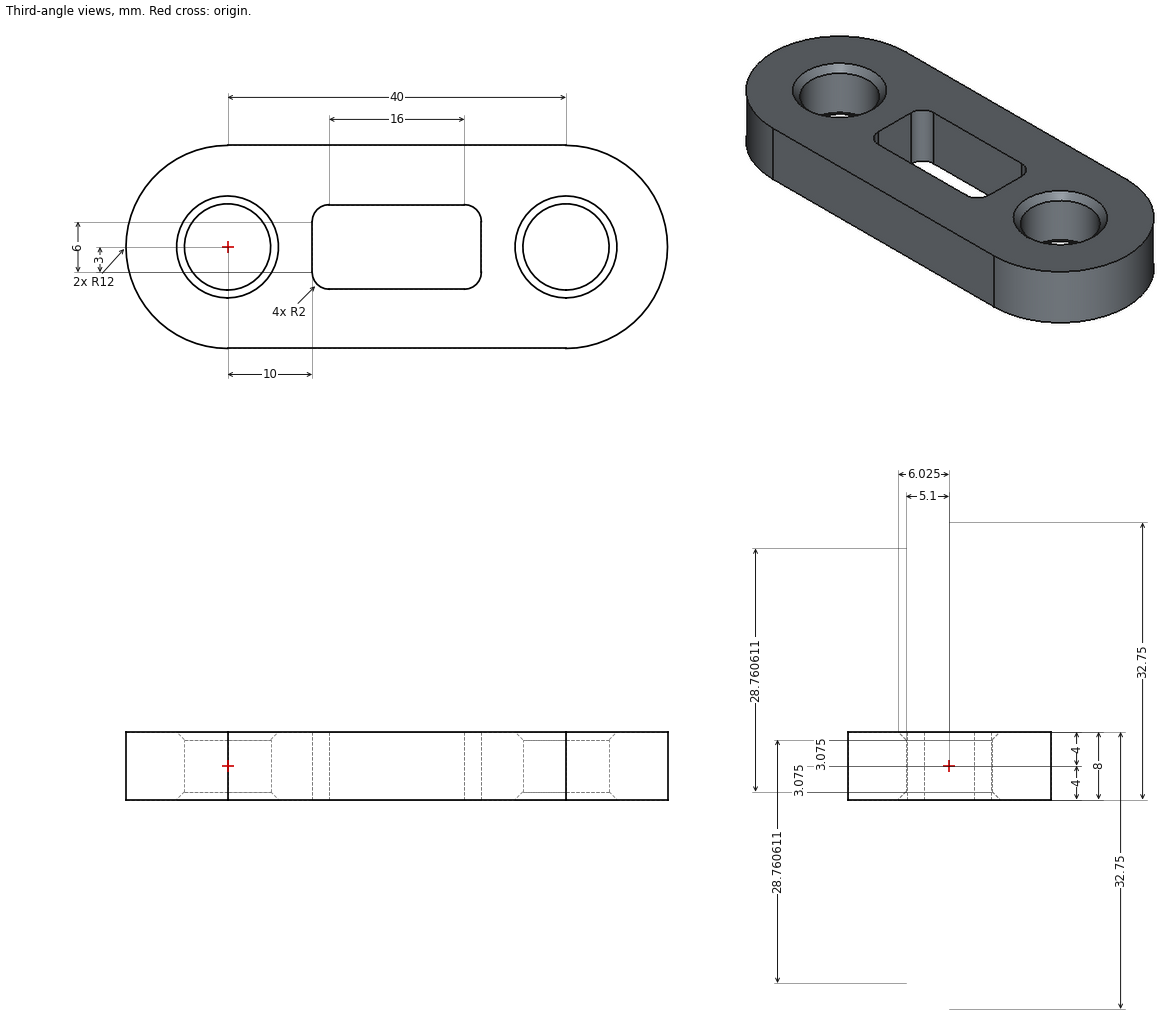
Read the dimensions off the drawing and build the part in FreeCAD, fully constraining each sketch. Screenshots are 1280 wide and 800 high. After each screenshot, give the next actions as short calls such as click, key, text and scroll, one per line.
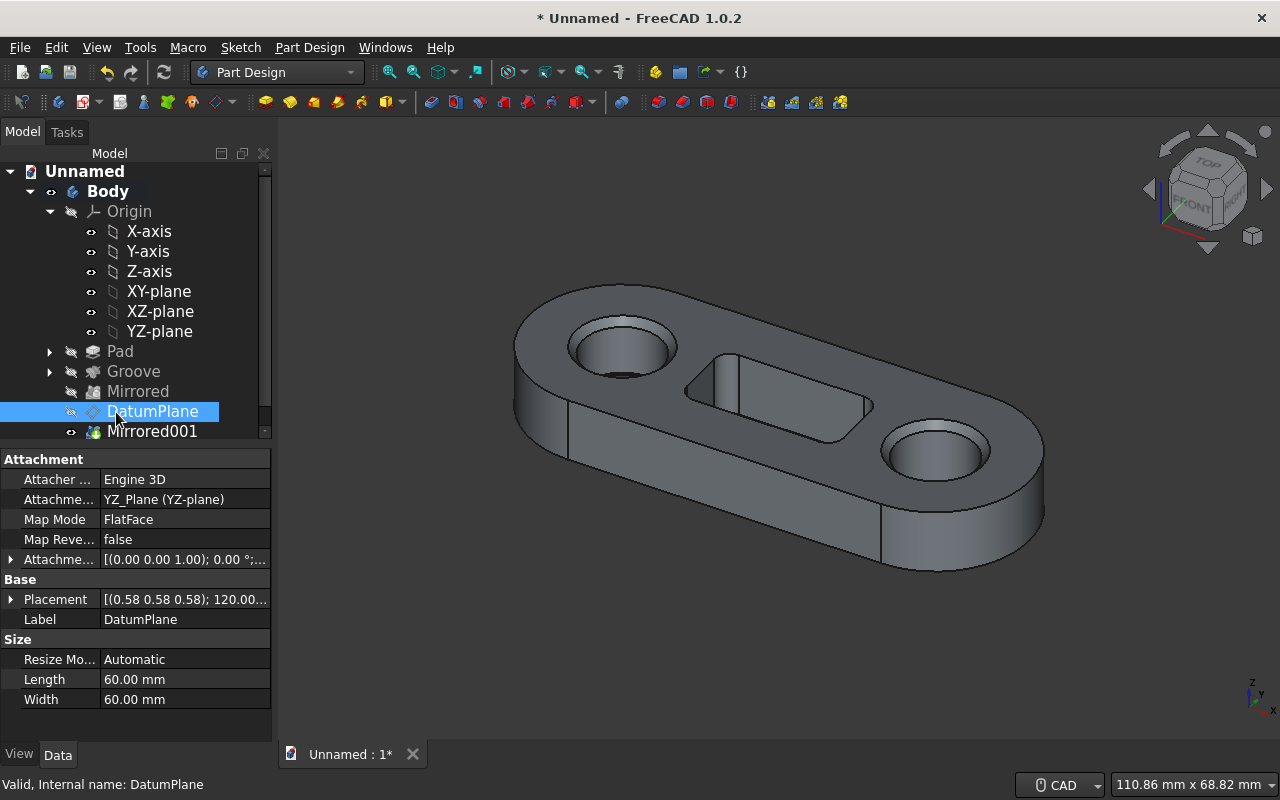
click(136, 332)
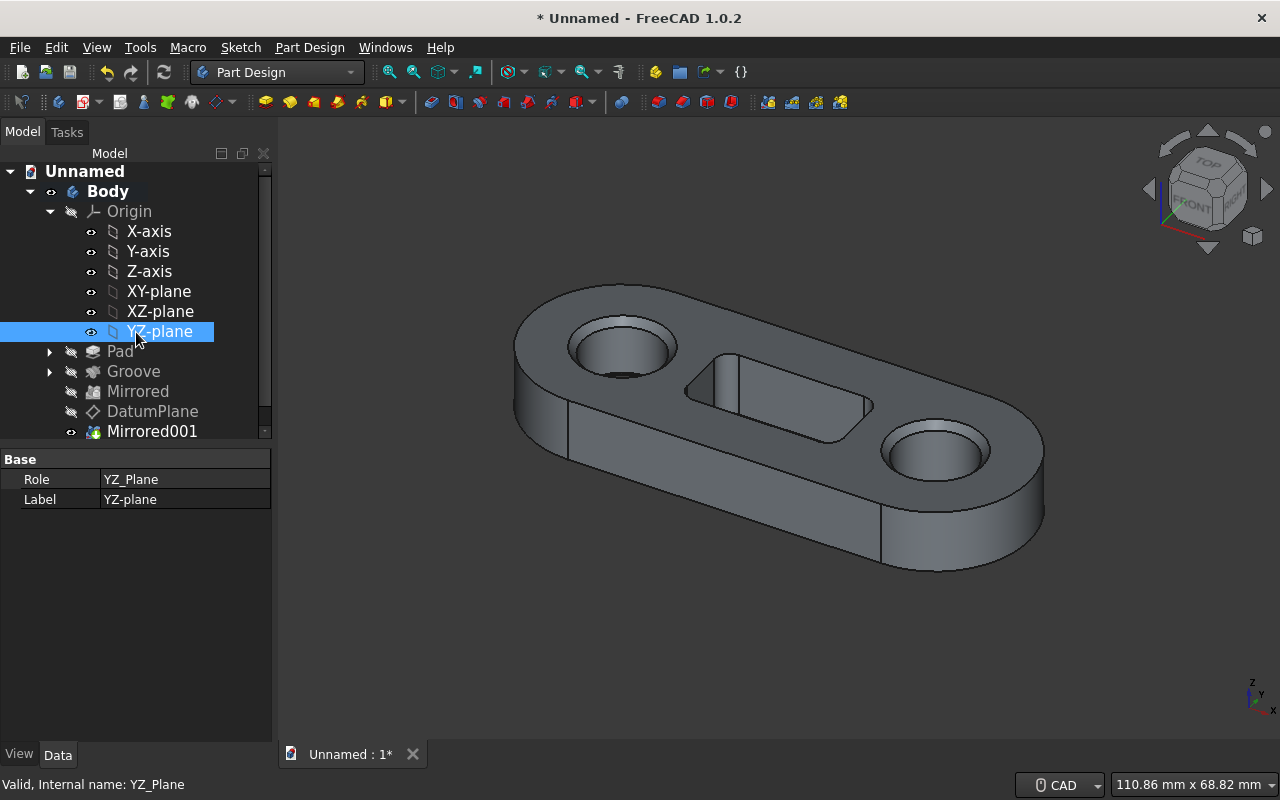
click(216, 102)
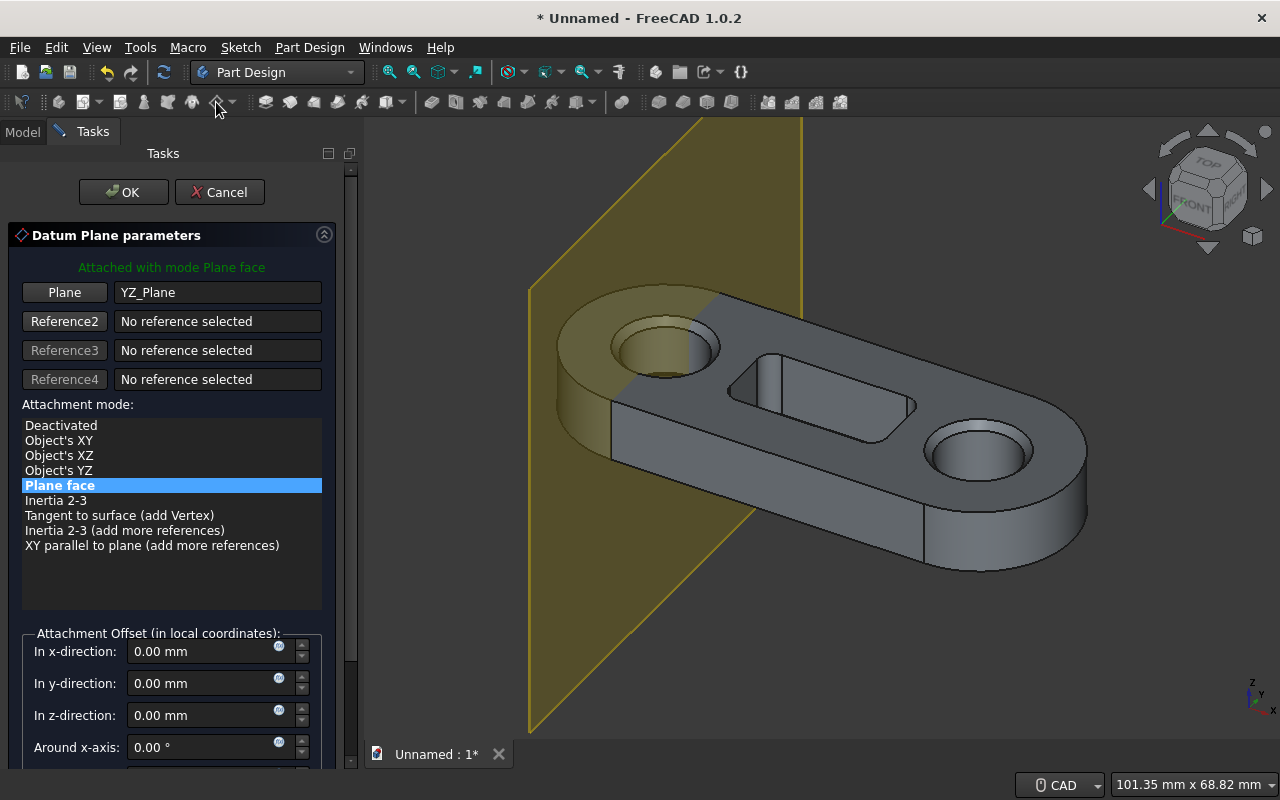
triple_click(210, 715)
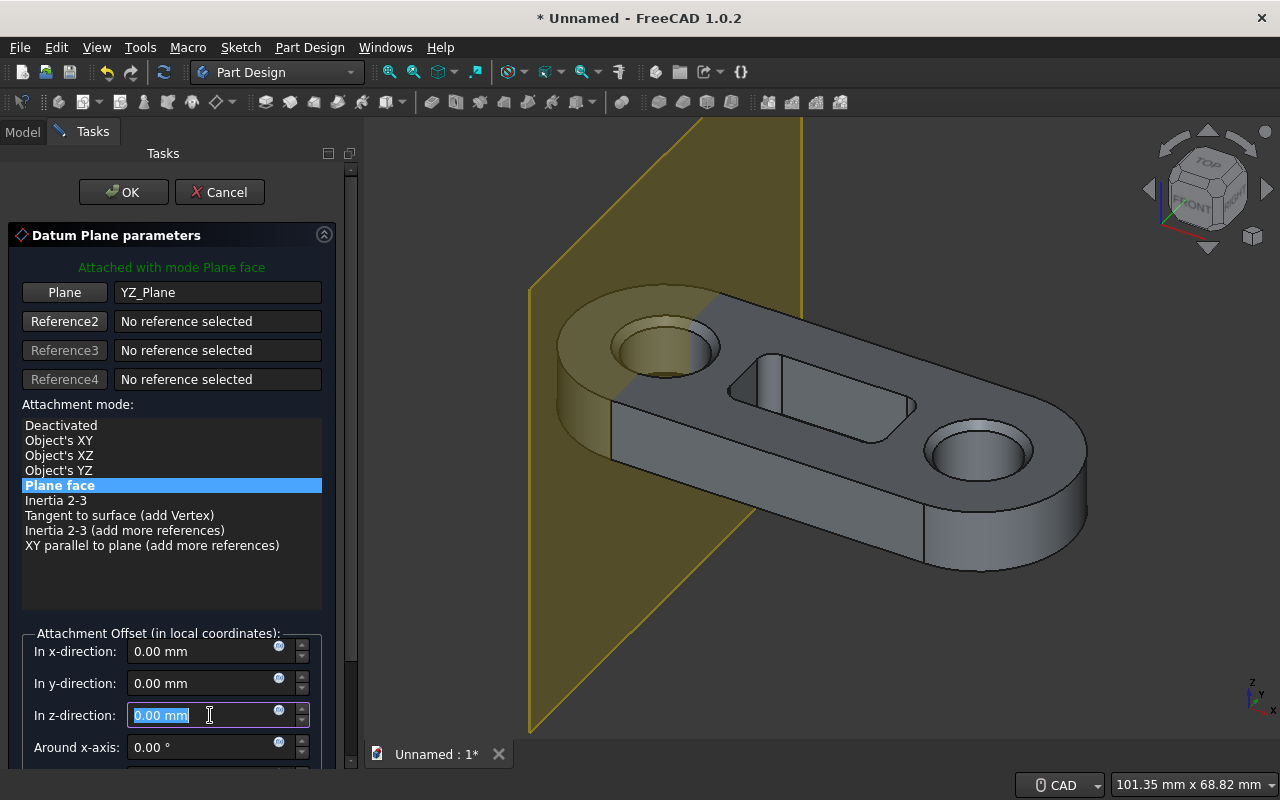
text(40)
key(Tab)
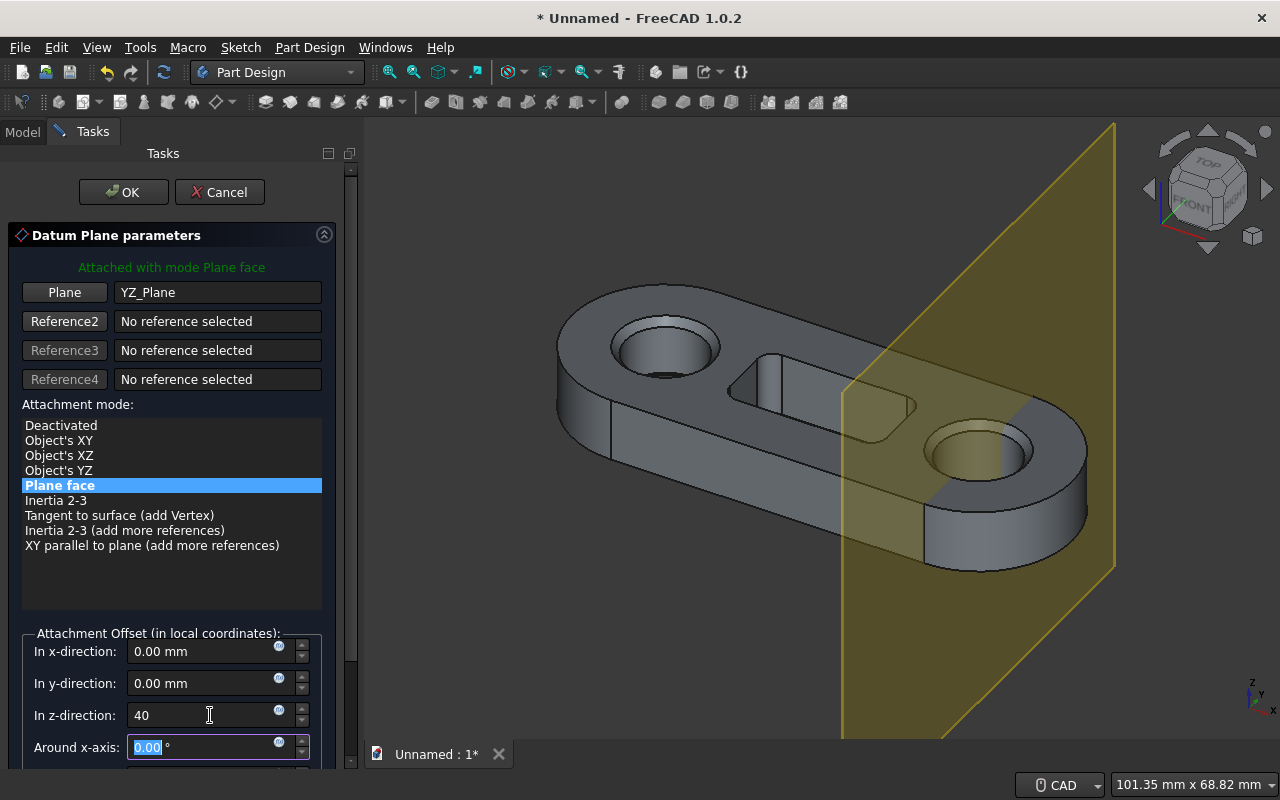
click(124, 192)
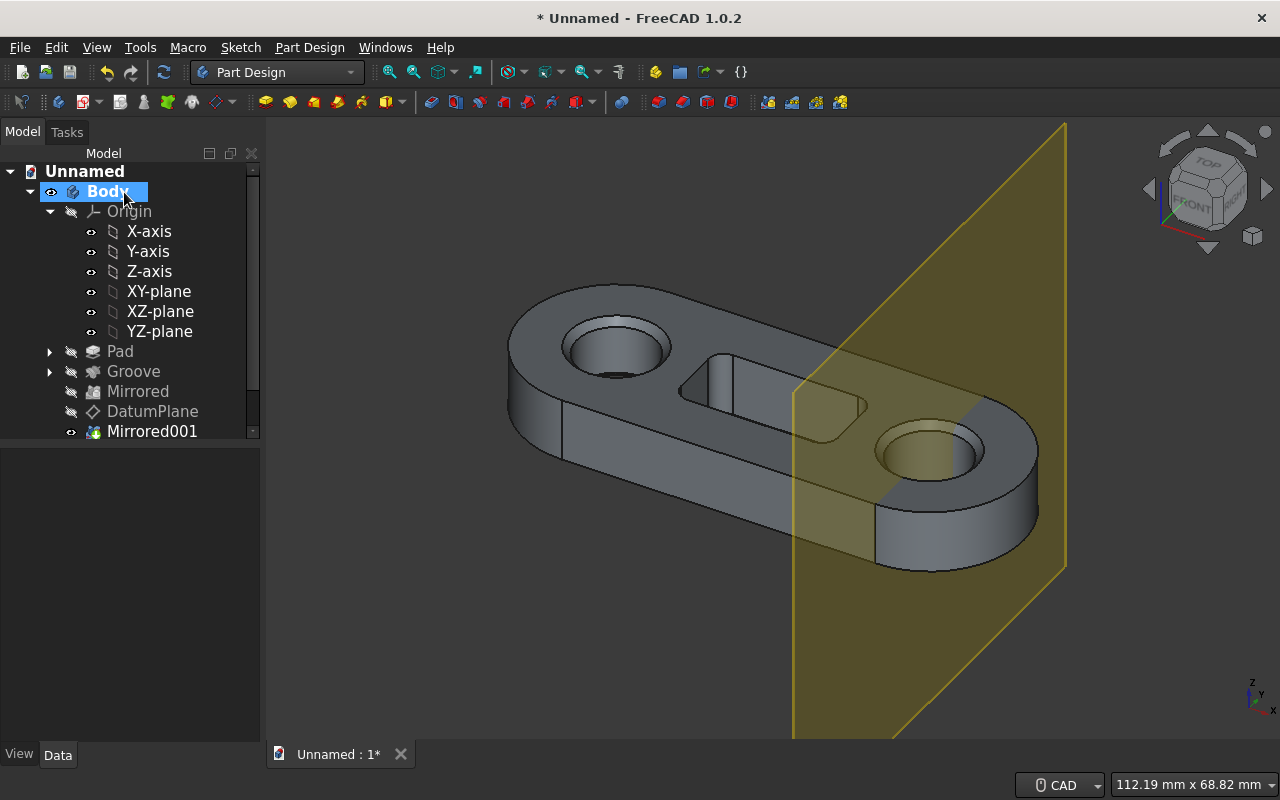
scroll(100, 307, down, 3)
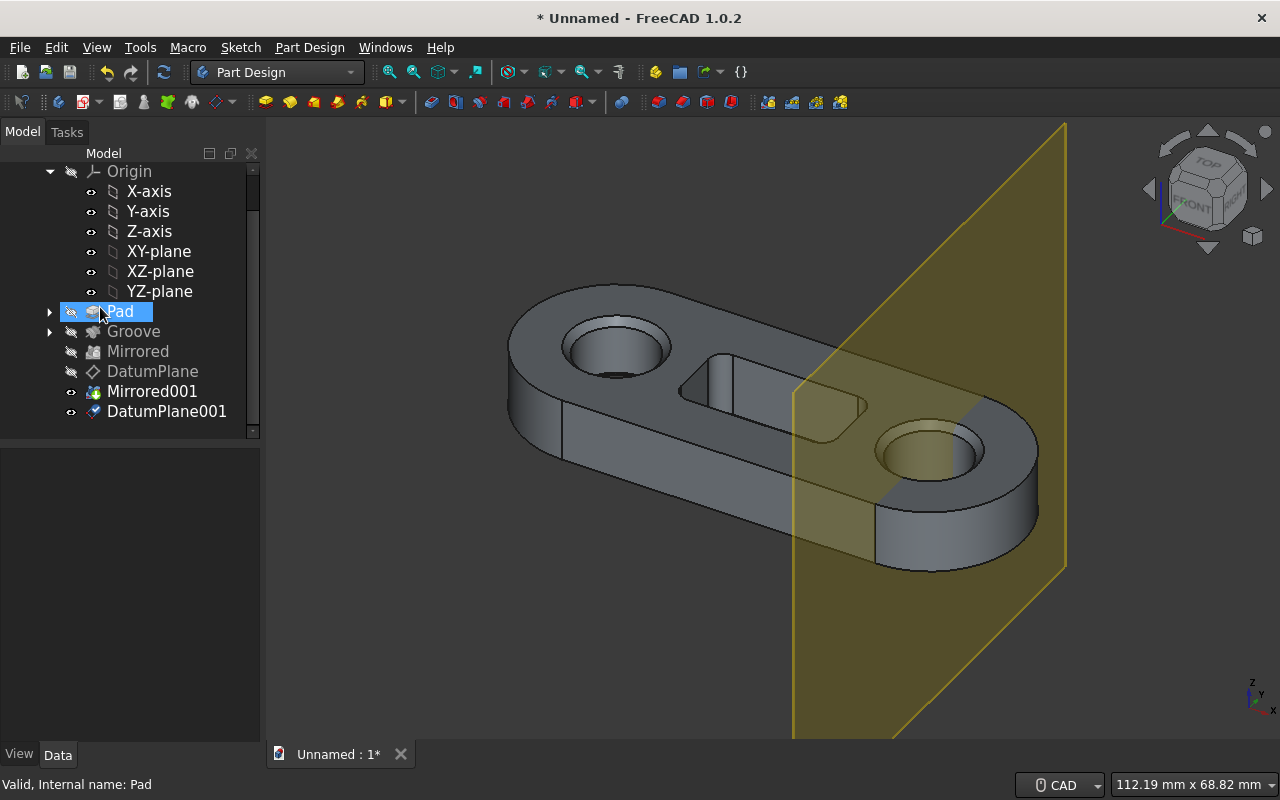
click(116, 412)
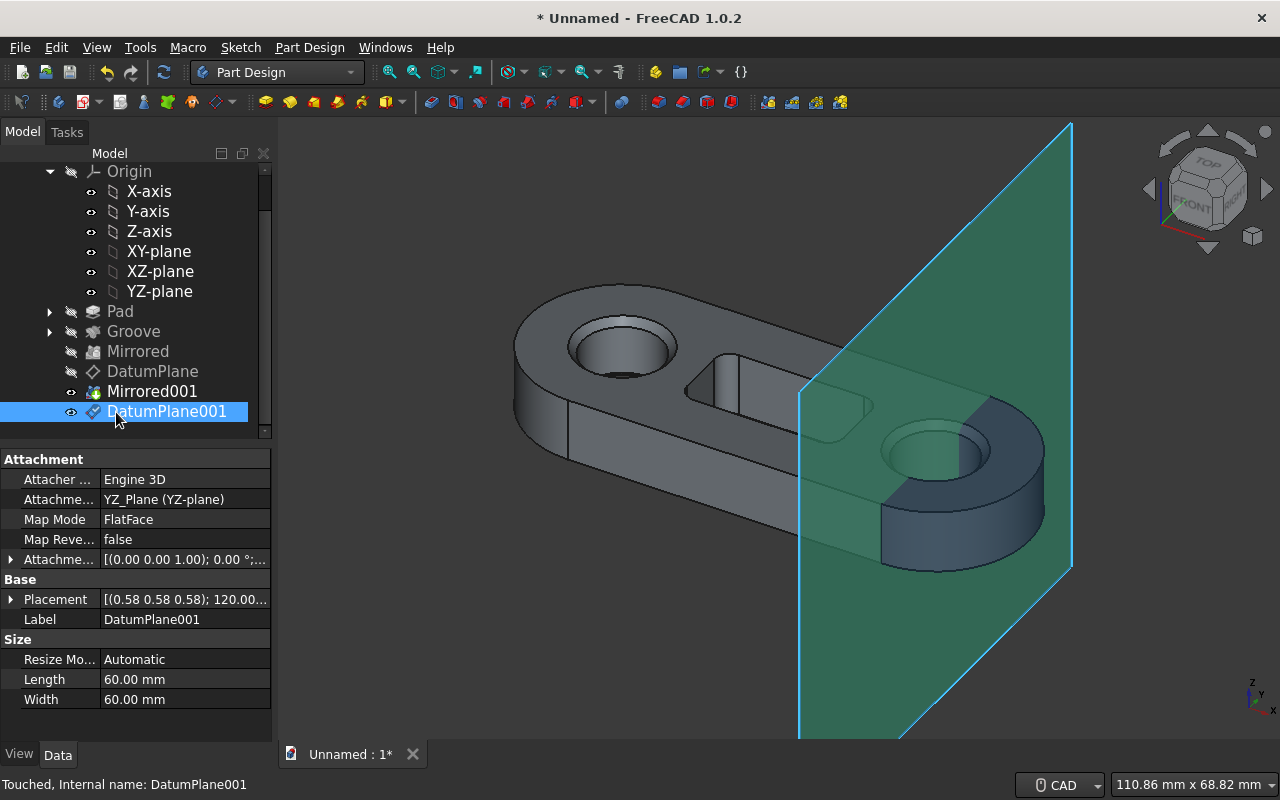
click(84, 102)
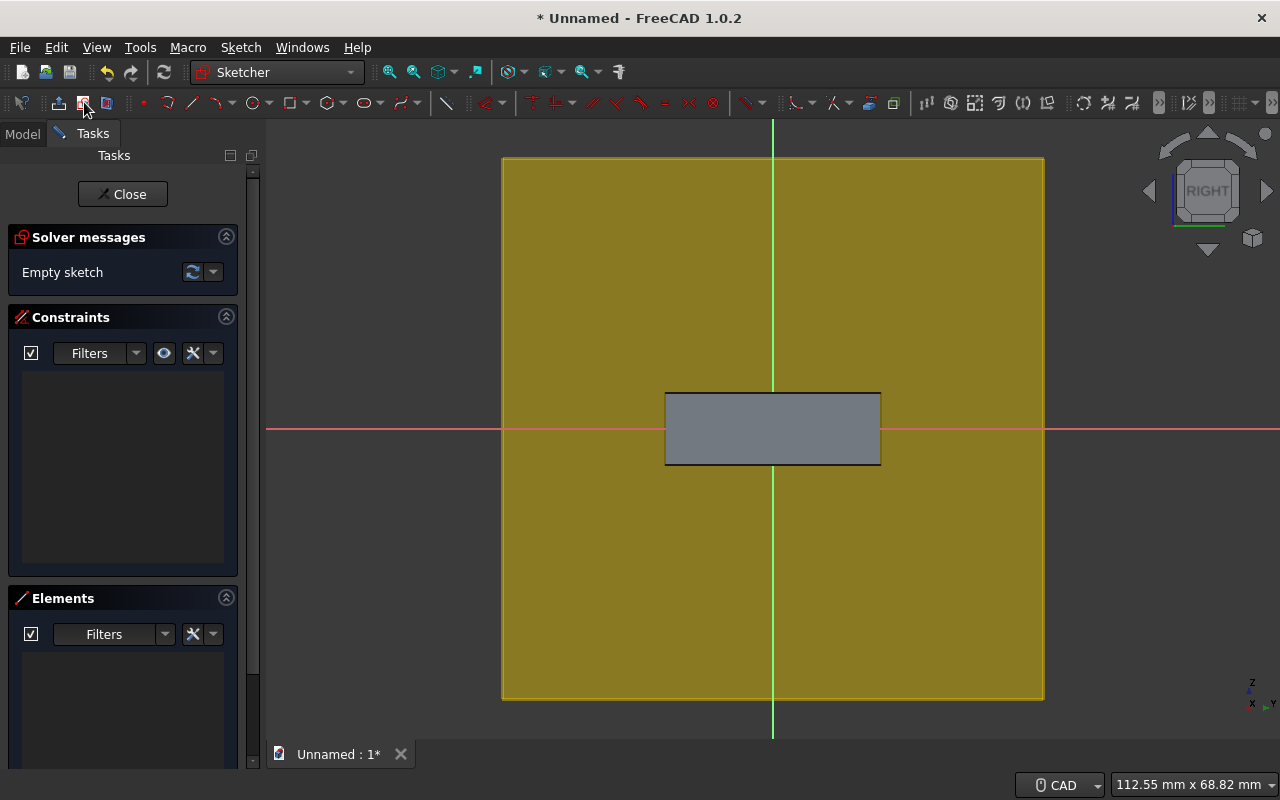
click(108, 104)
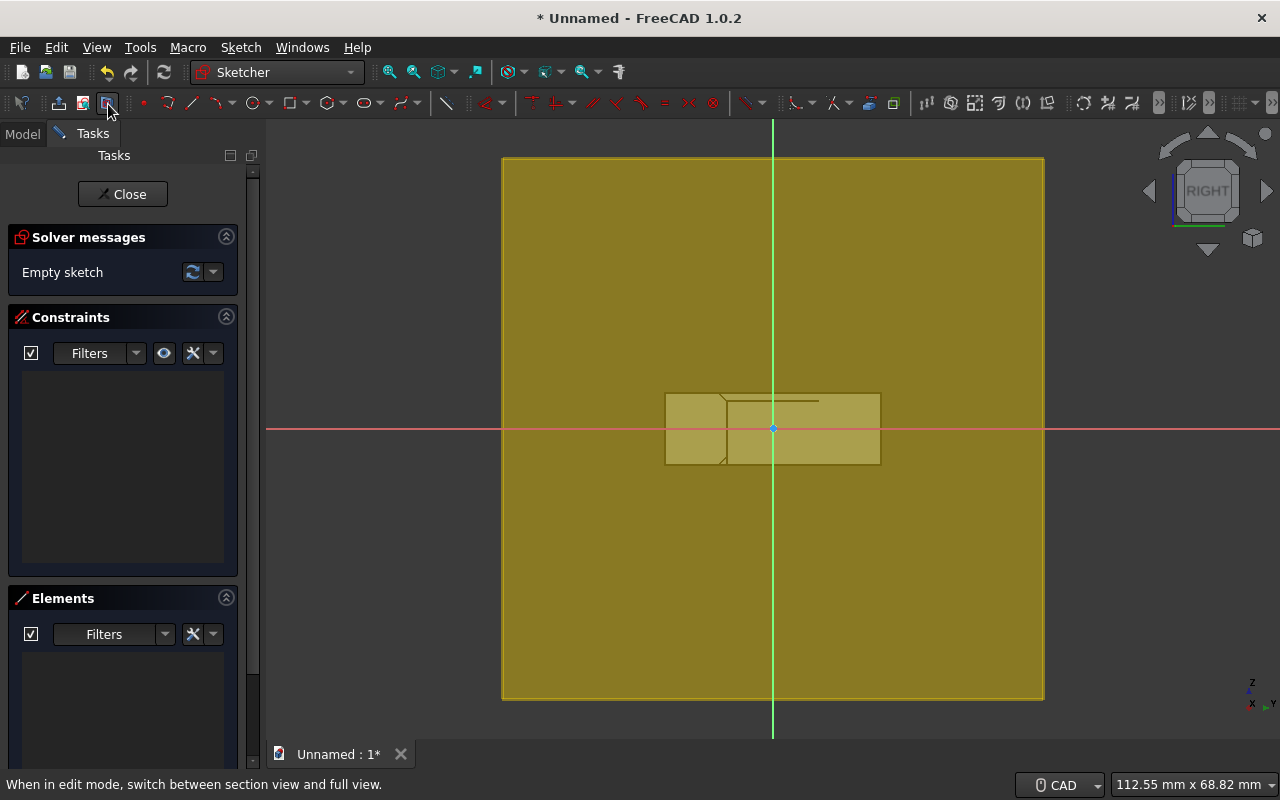
scroll(933, 147, up, 1)